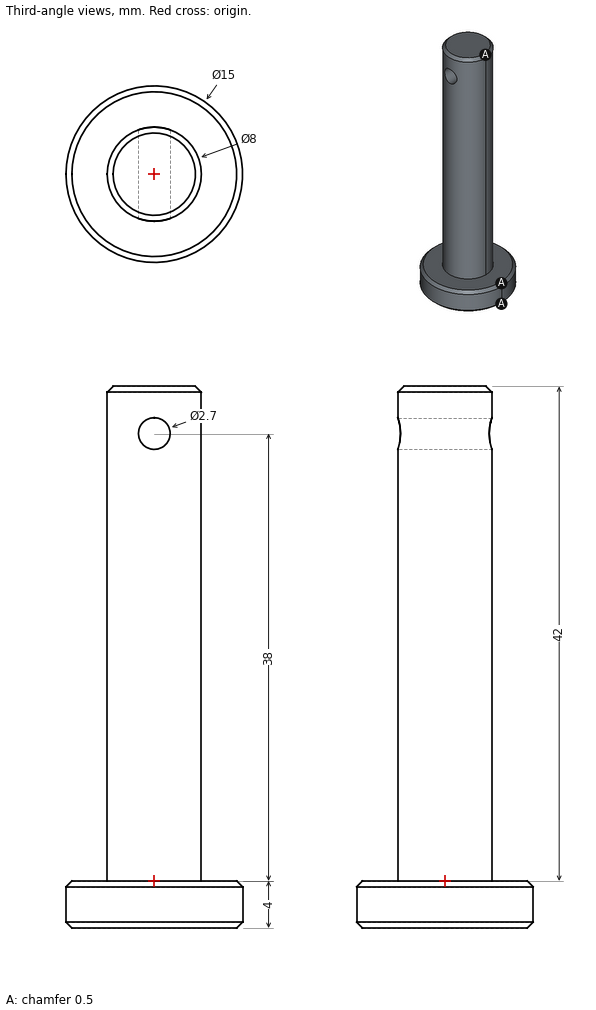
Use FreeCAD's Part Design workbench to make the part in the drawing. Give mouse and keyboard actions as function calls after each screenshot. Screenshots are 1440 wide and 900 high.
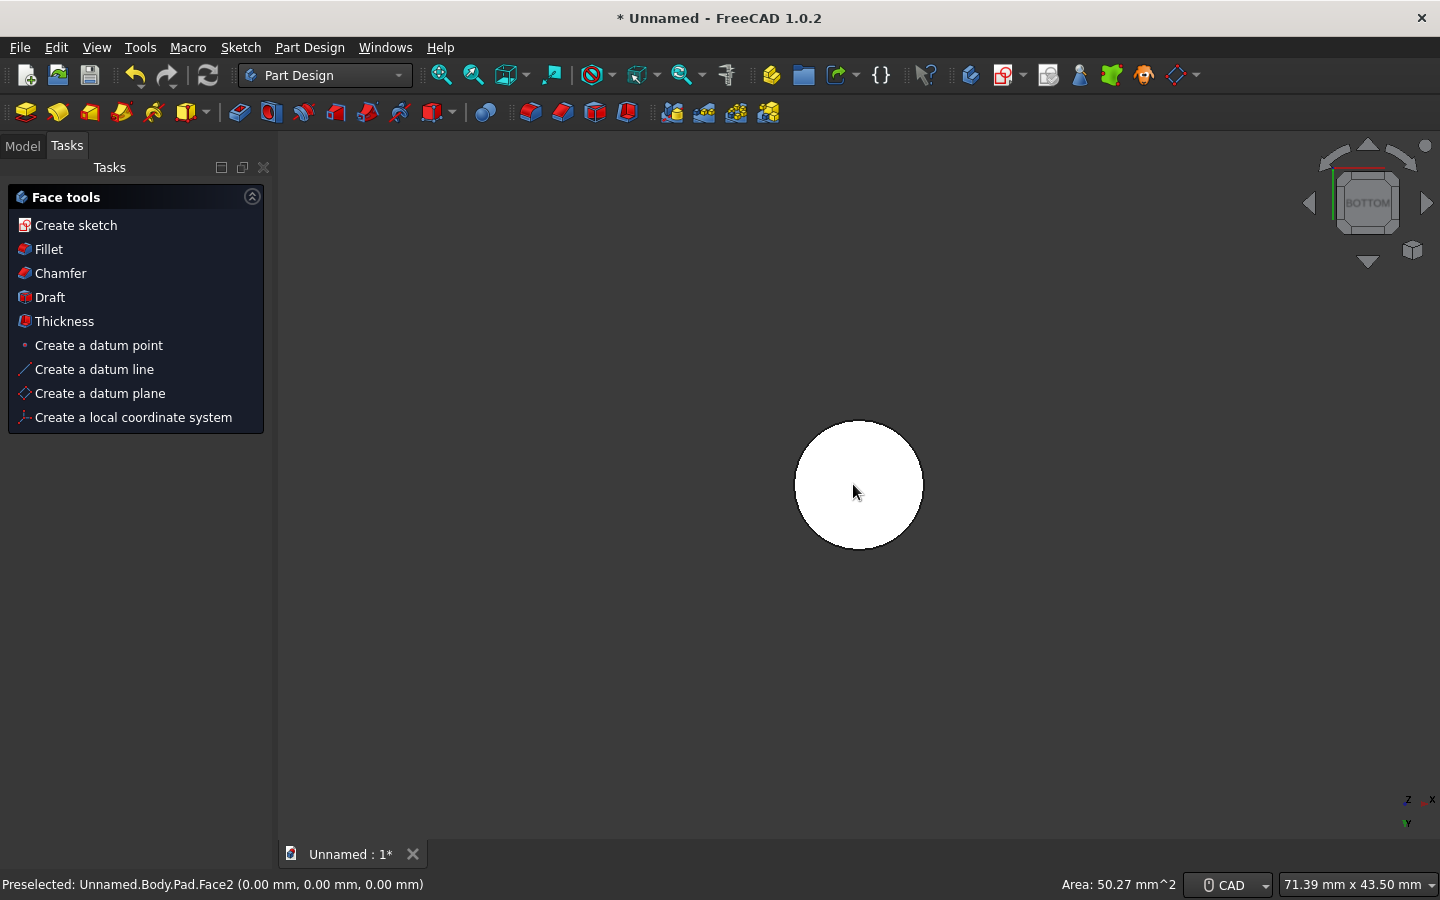
click(1004, 76)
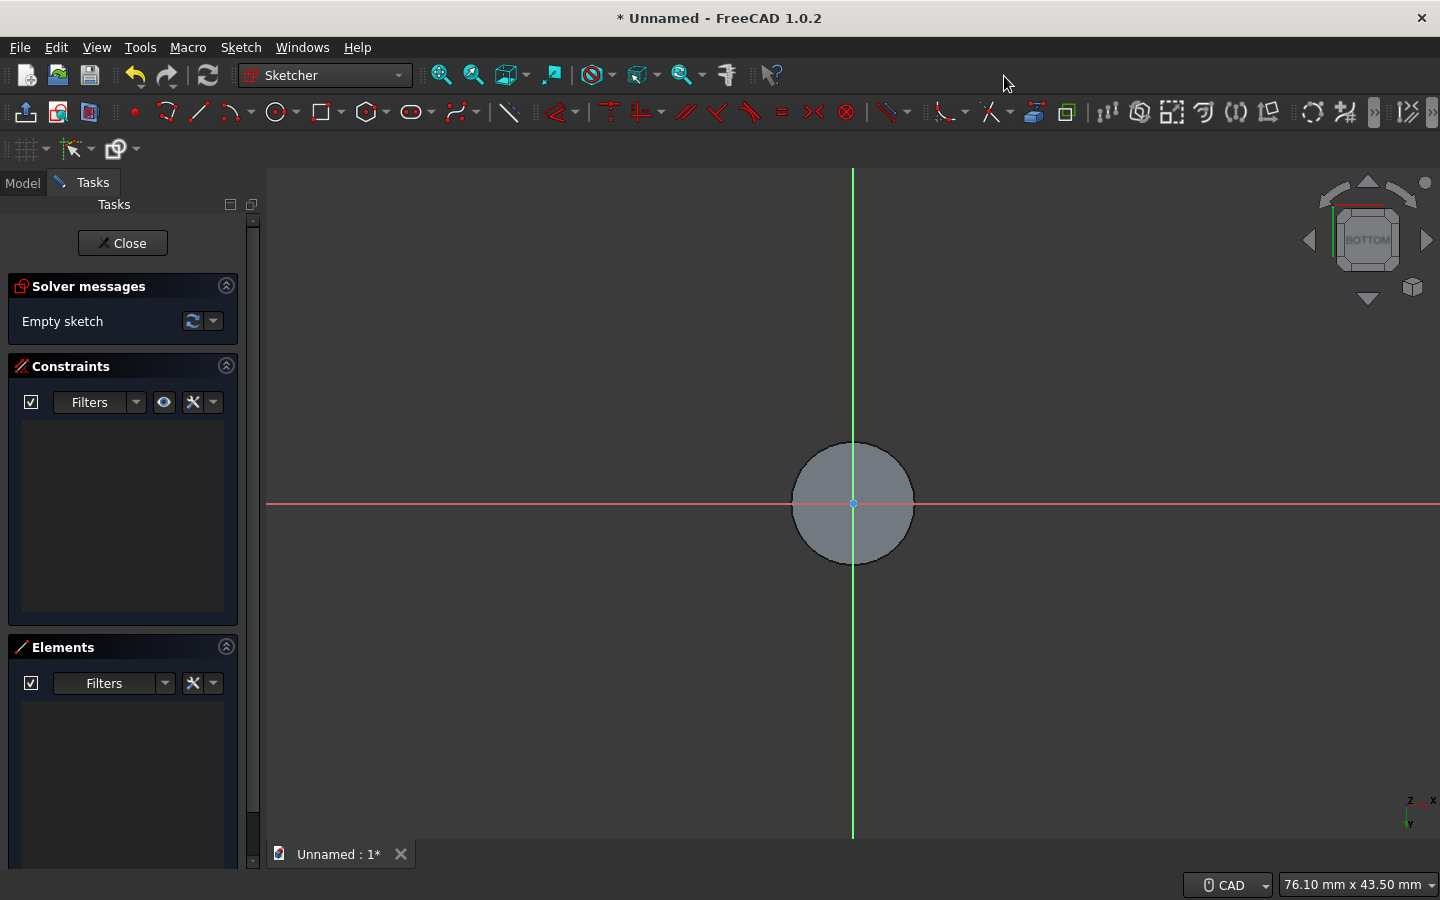
scroll(936, 504, up, 3)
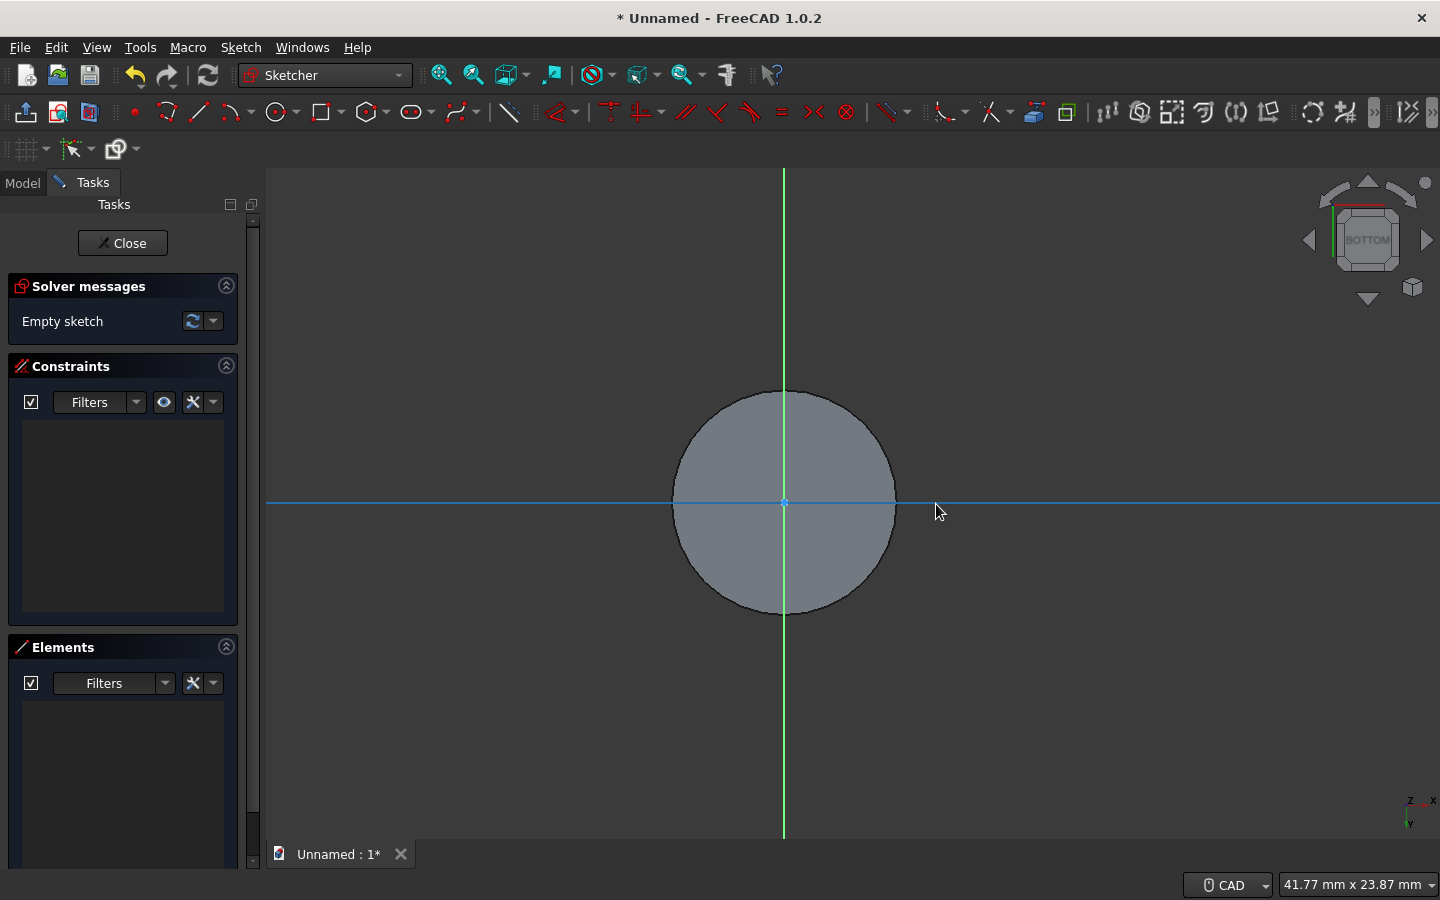
click(276, 112)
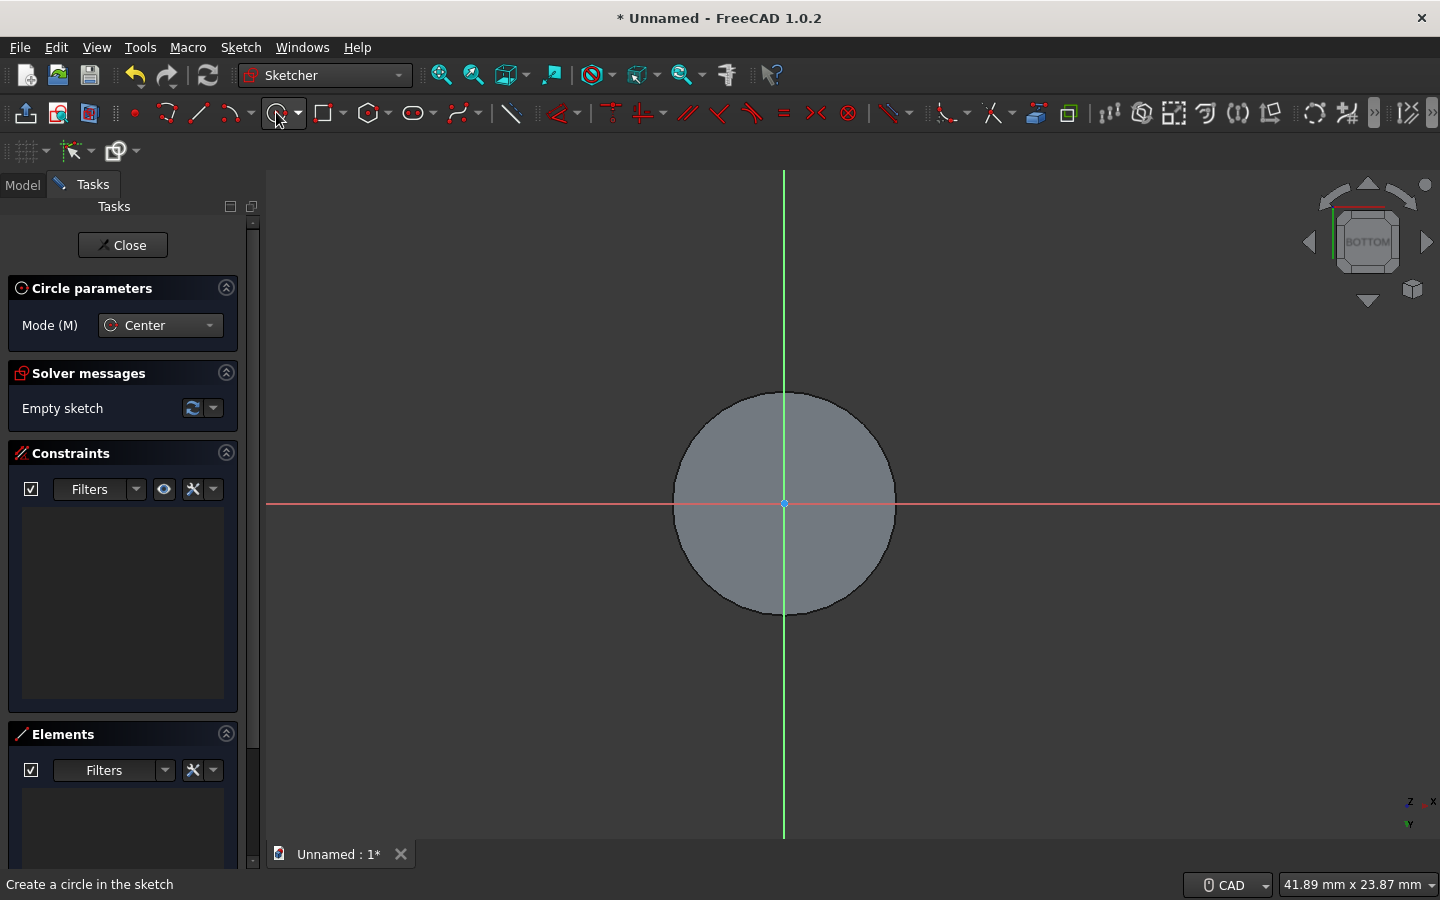
click(784, 504)
move(933, 355)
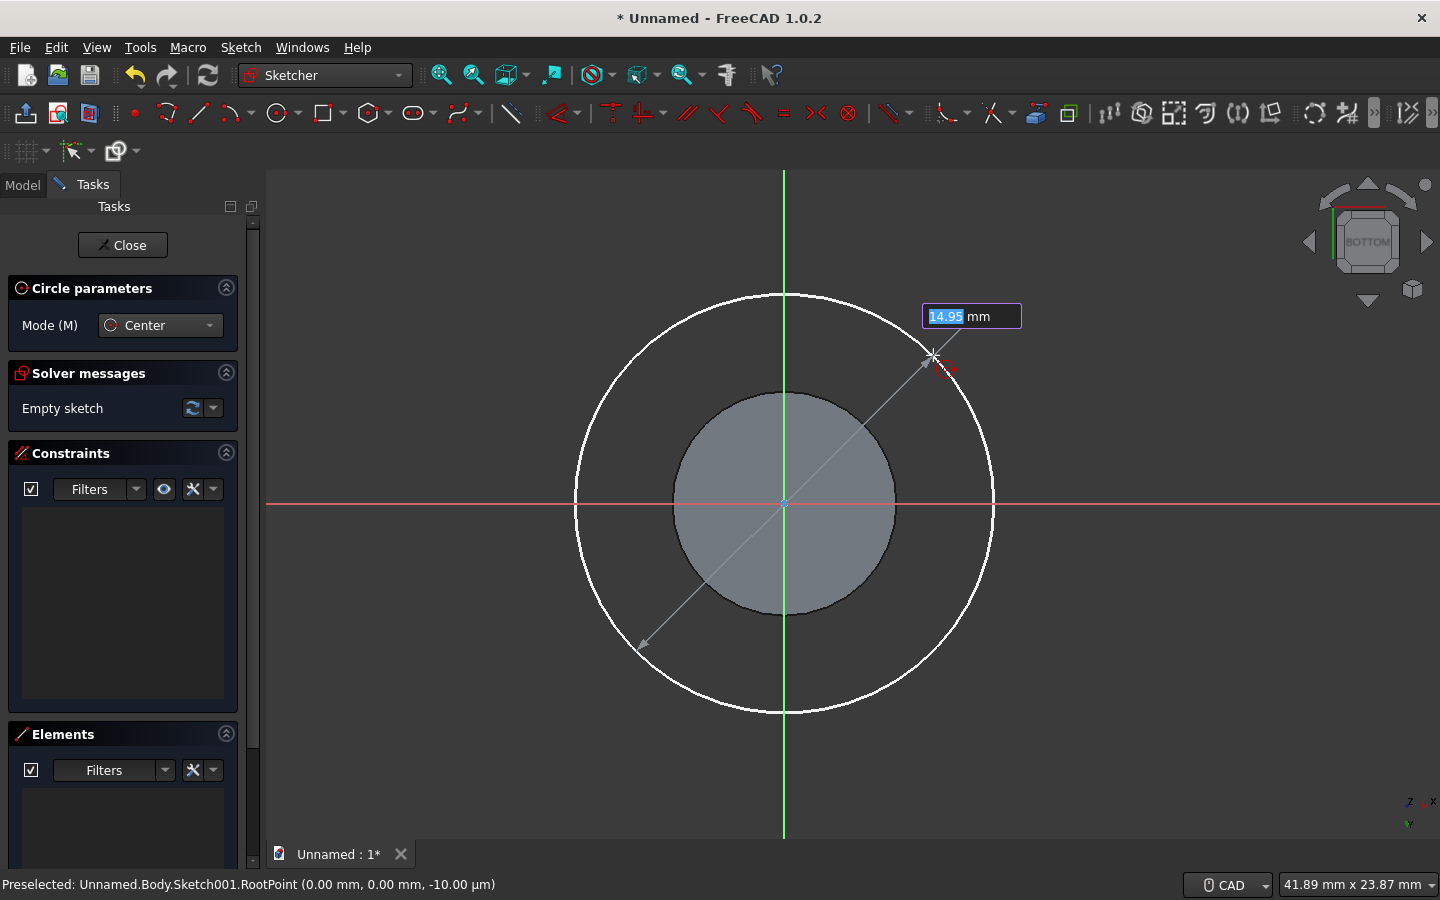
text(15)
key(Return)
key(Escape)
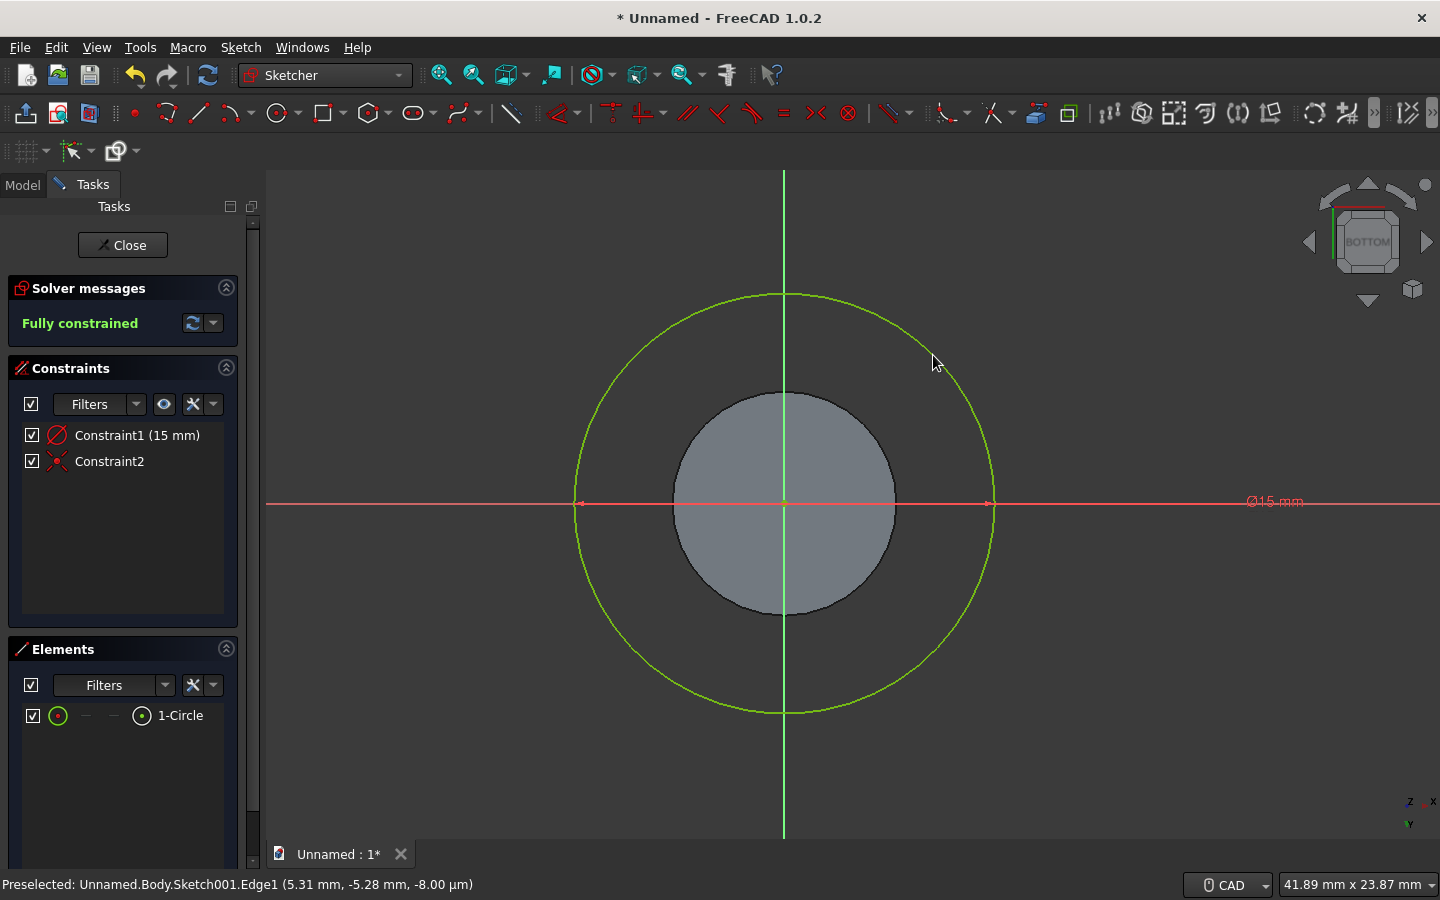
click(123, 245)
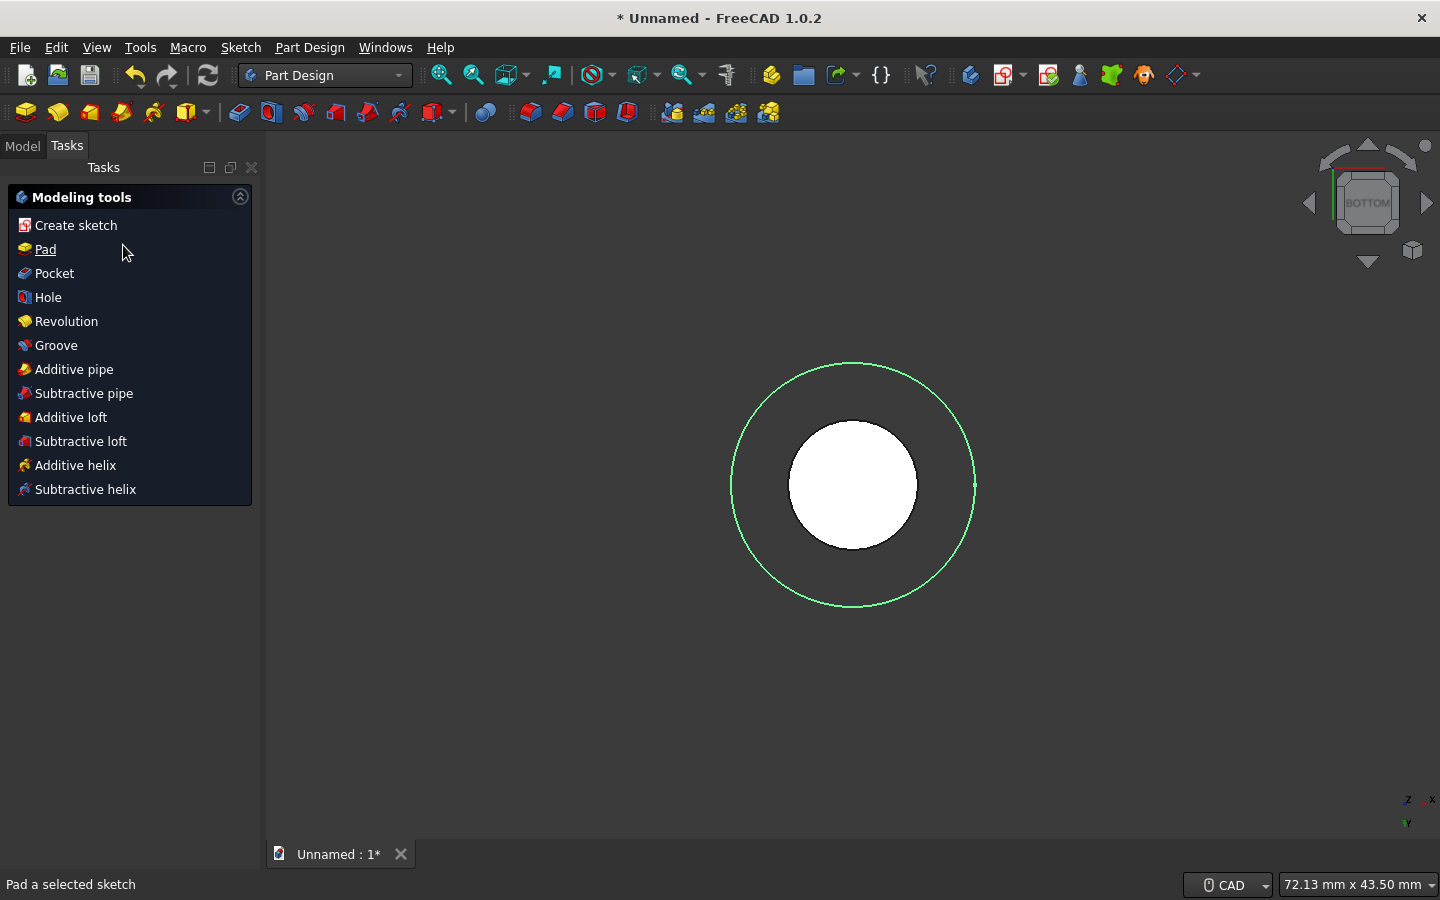
click(26, 112)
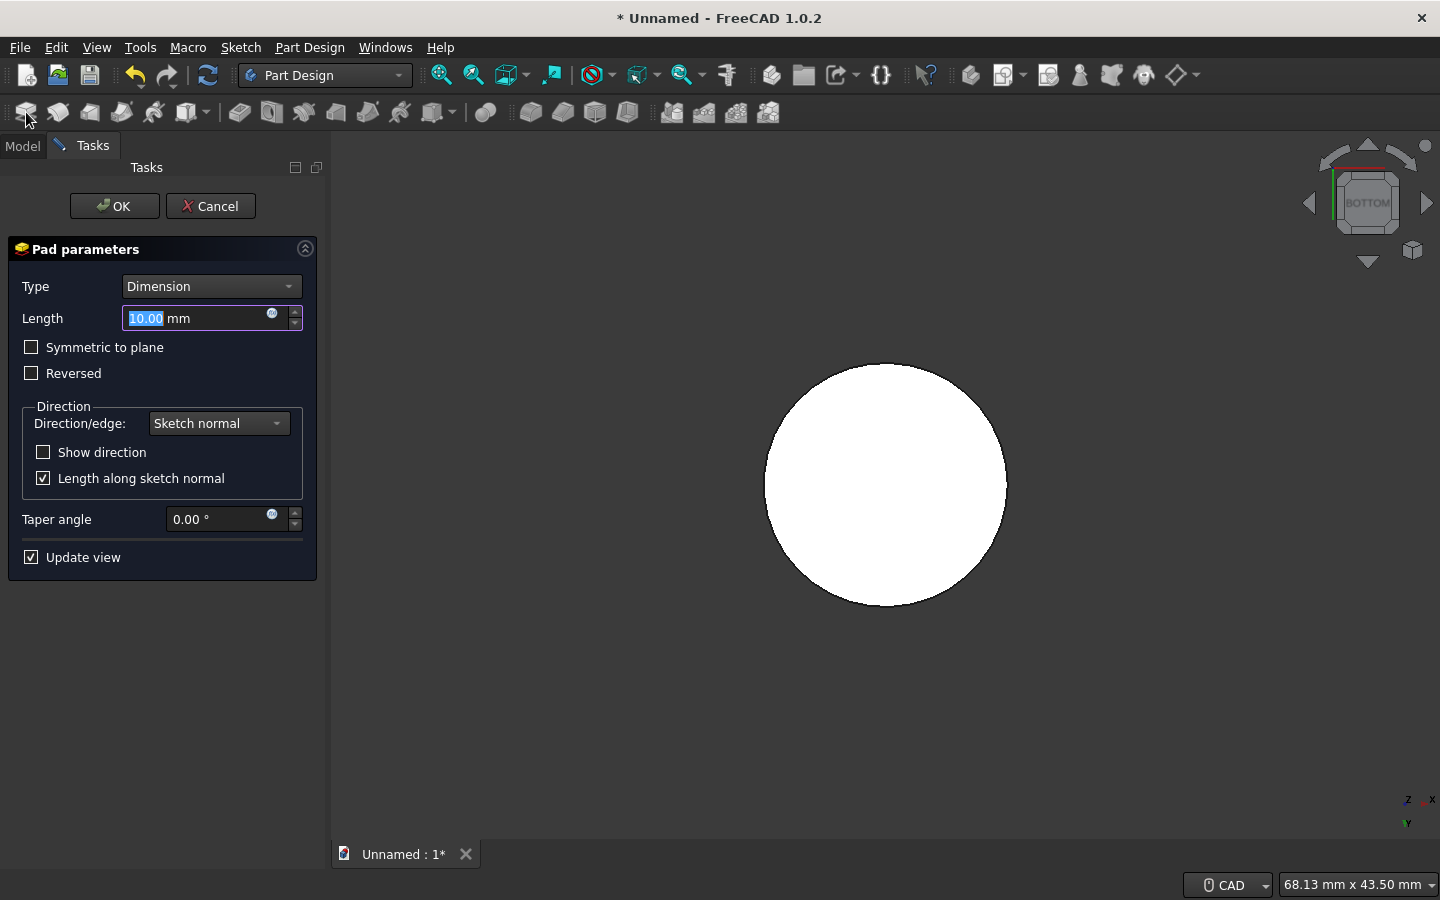
text(4)
key(Tab)